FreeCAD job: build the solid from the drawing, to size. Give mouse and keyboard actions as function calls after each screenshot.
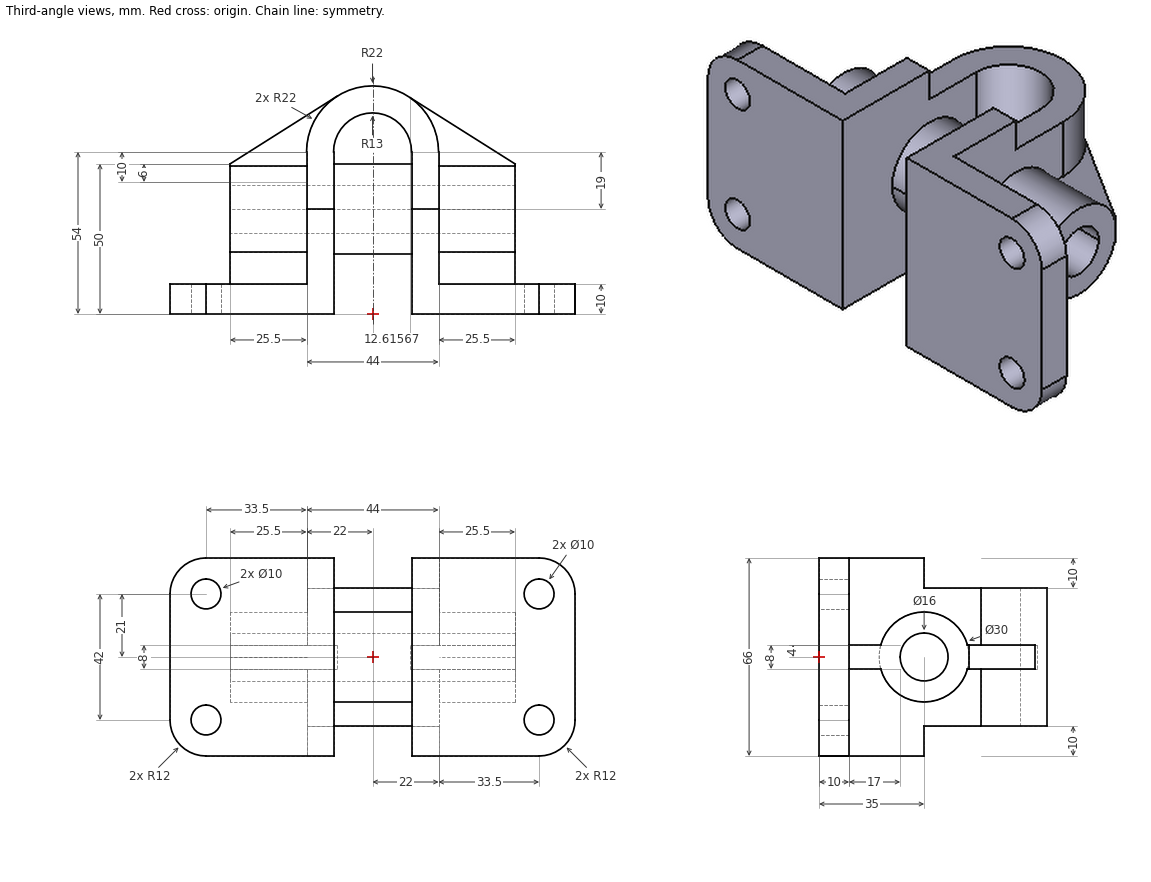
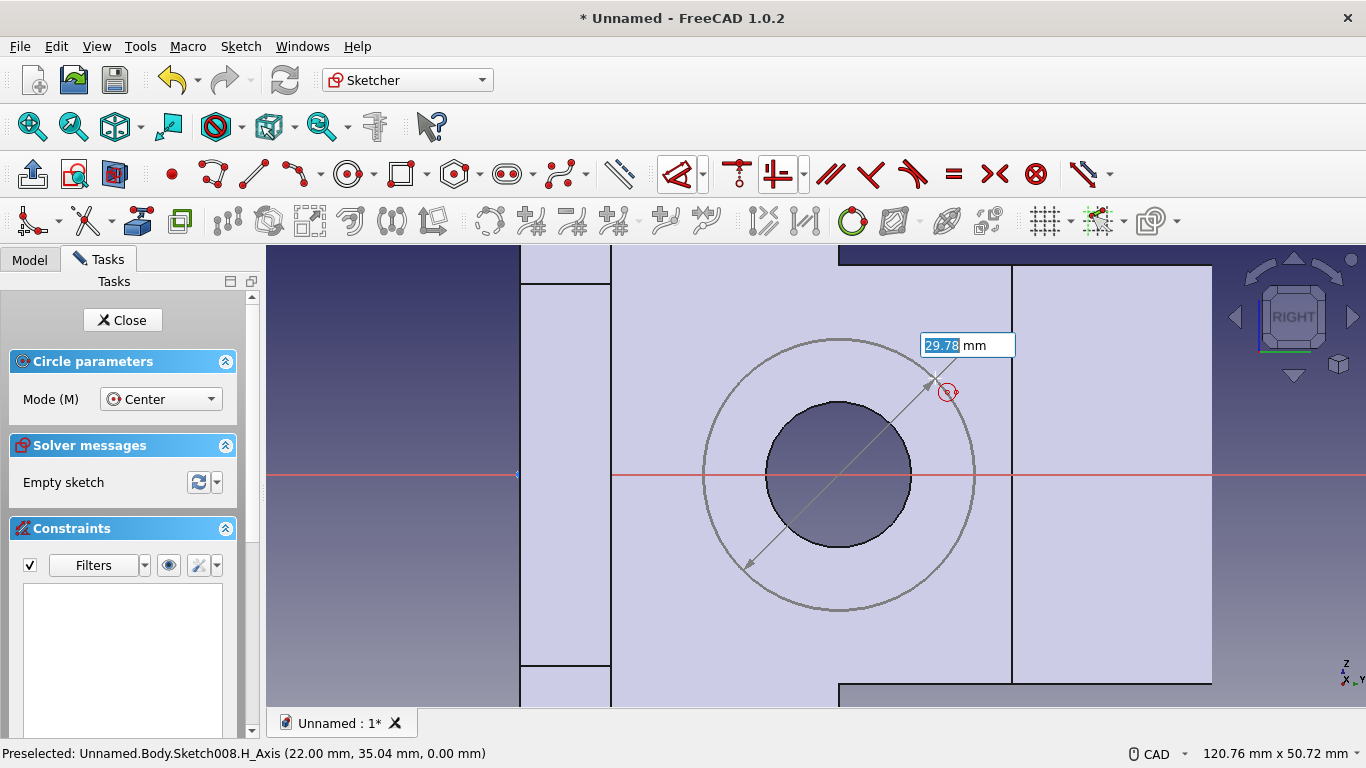
text(30)
key(Return)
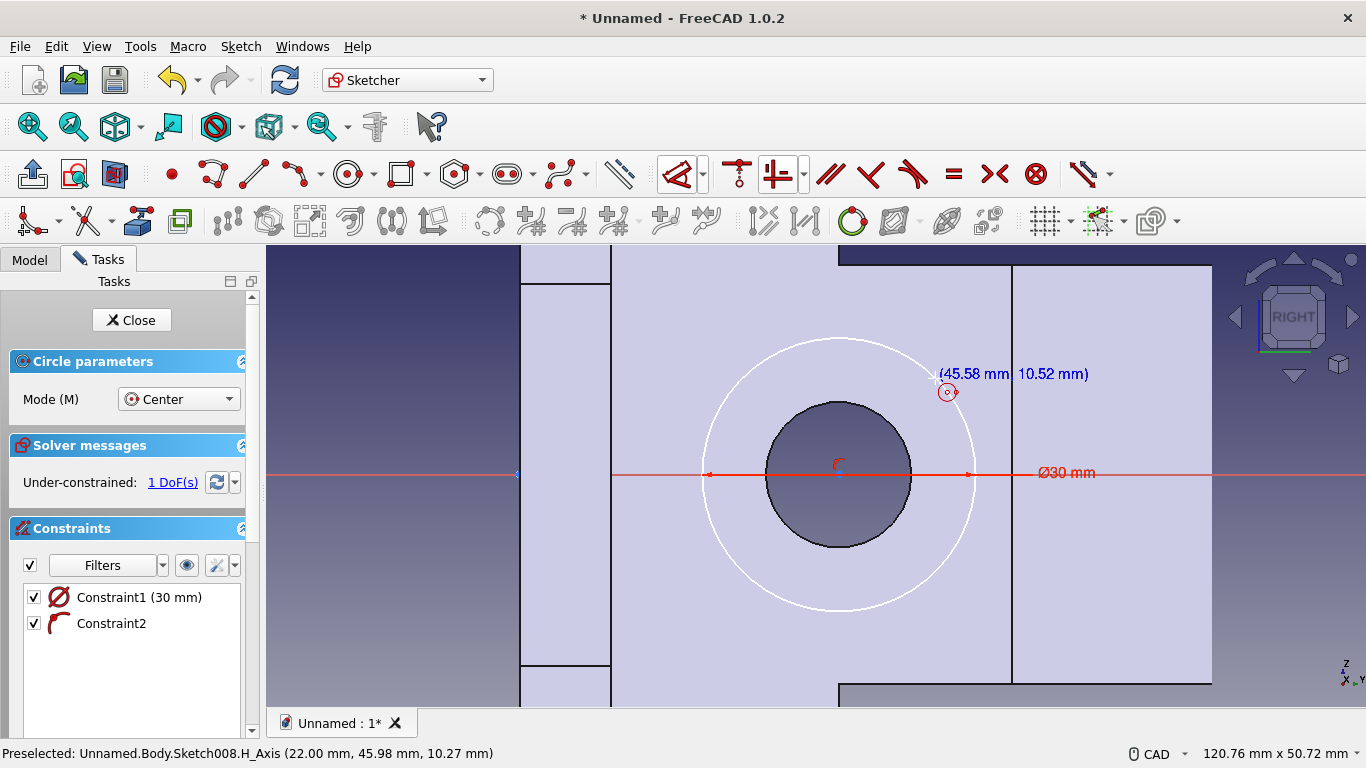
click(839, 475)
move(890, 423)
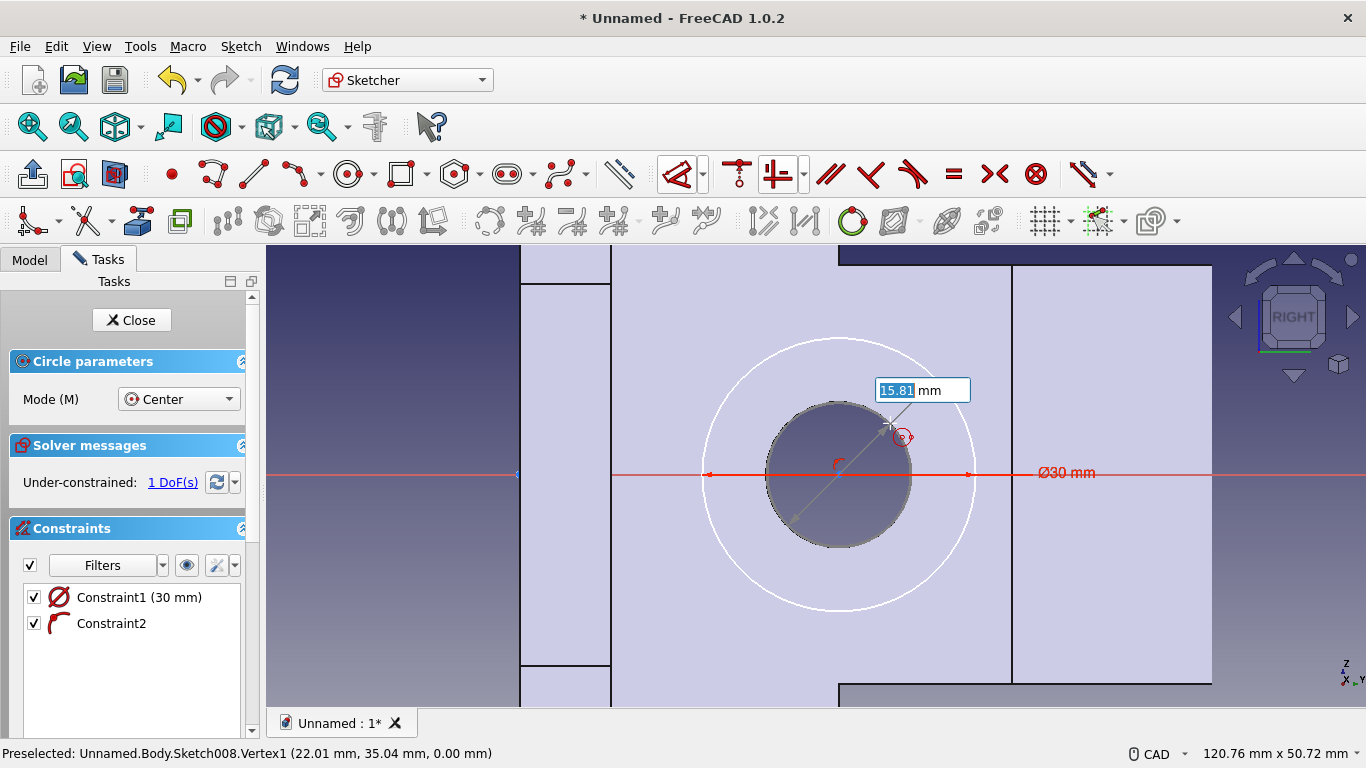
text(16)
key(Return)
key(Escape)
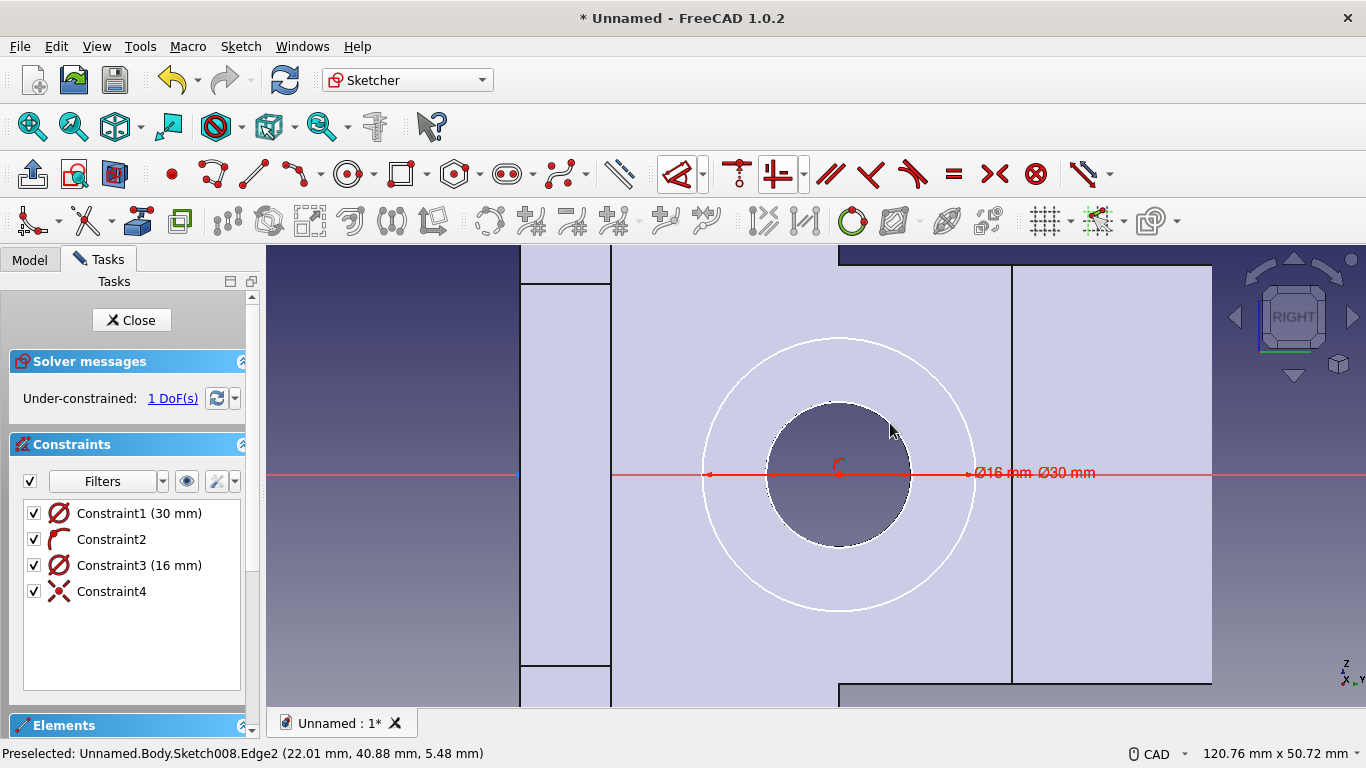
click(839, 475)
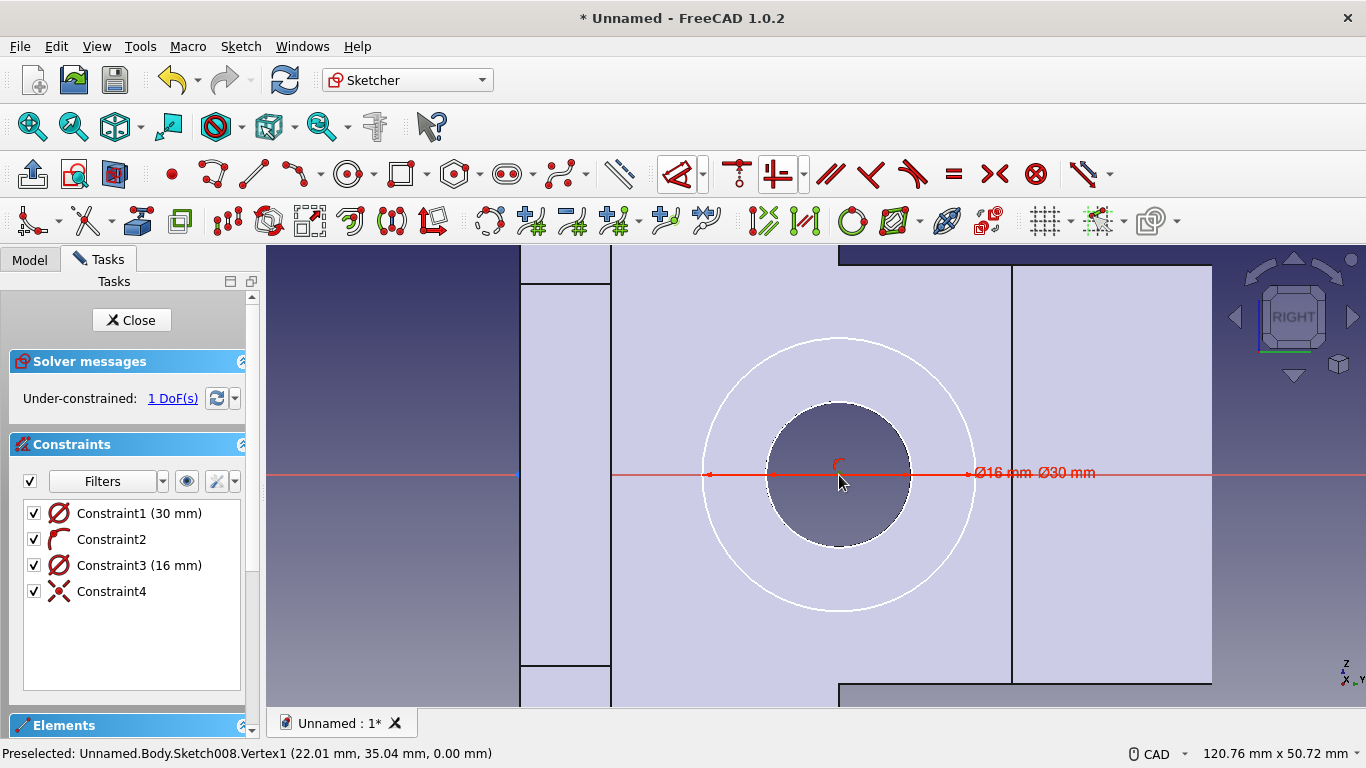
key(l)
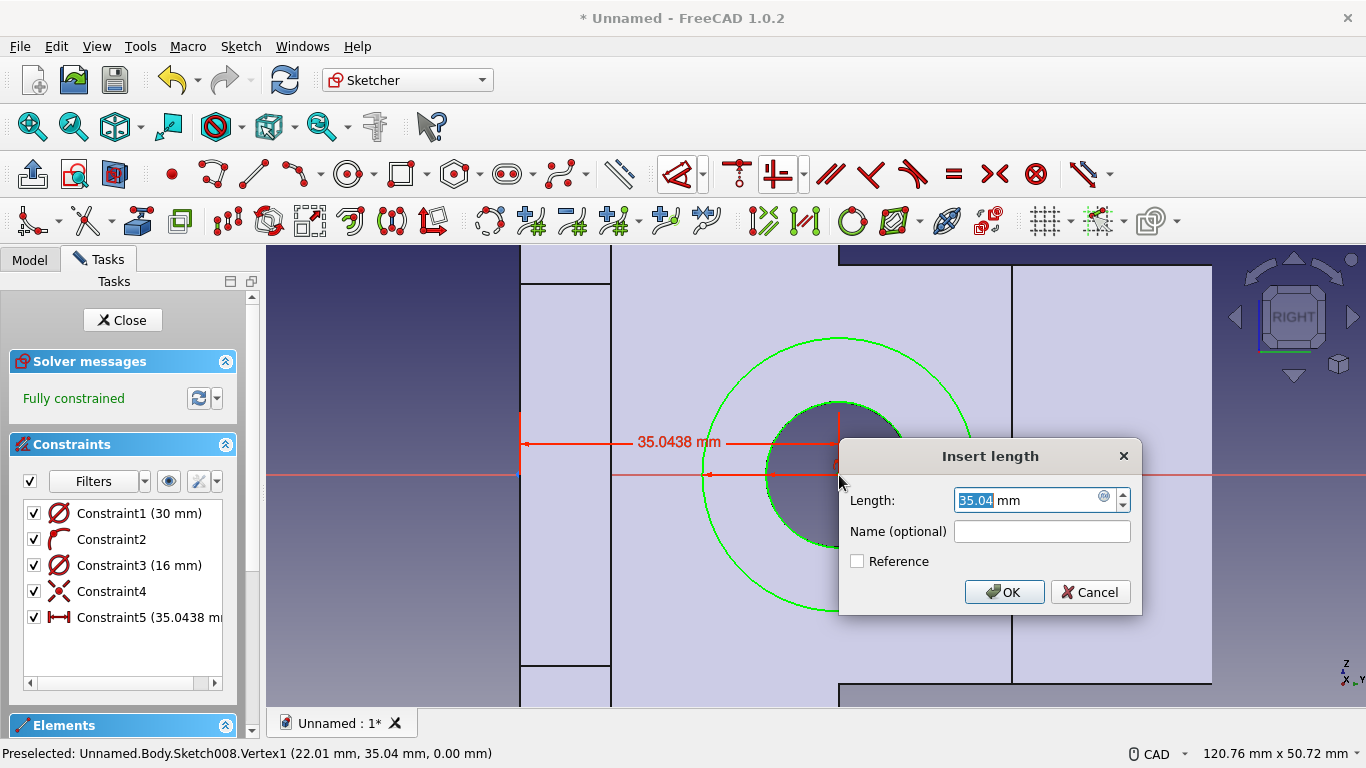
text(35)
key(Return)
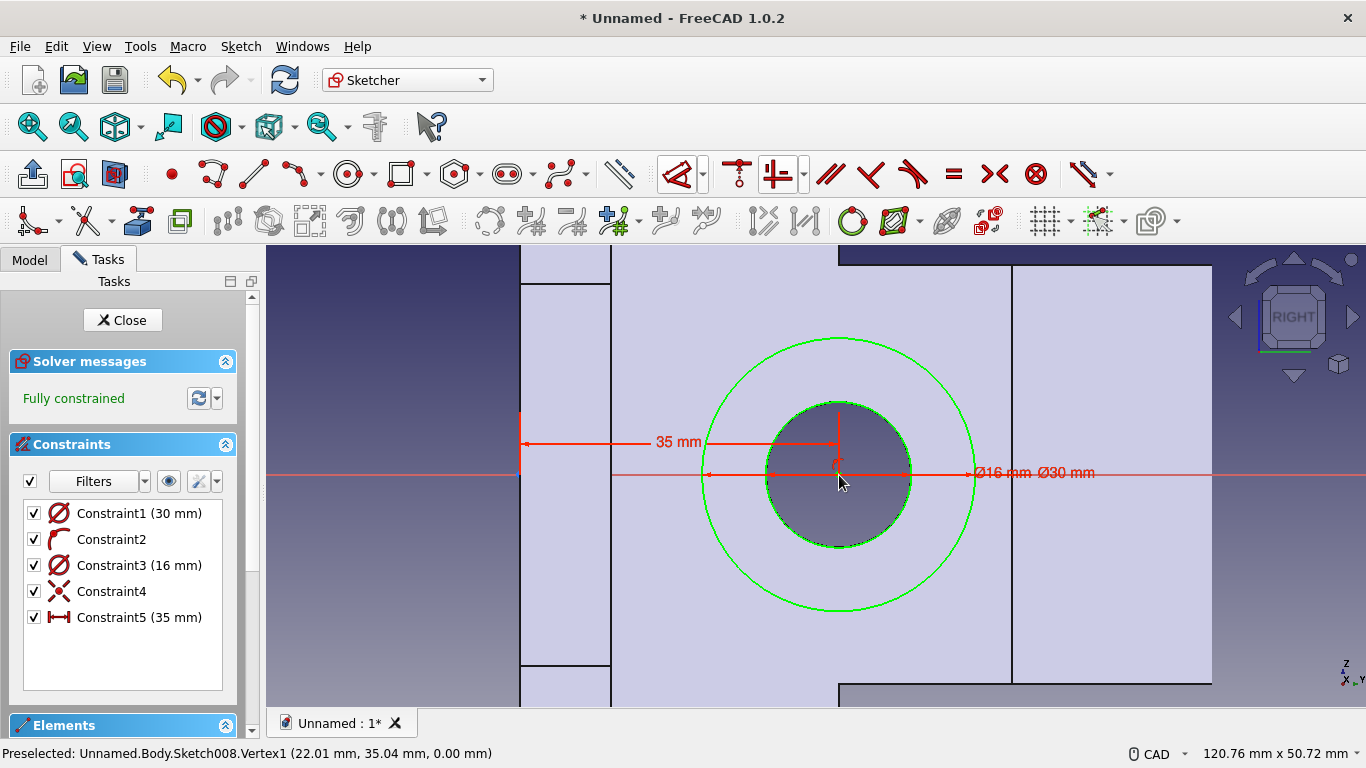
click(123, 320)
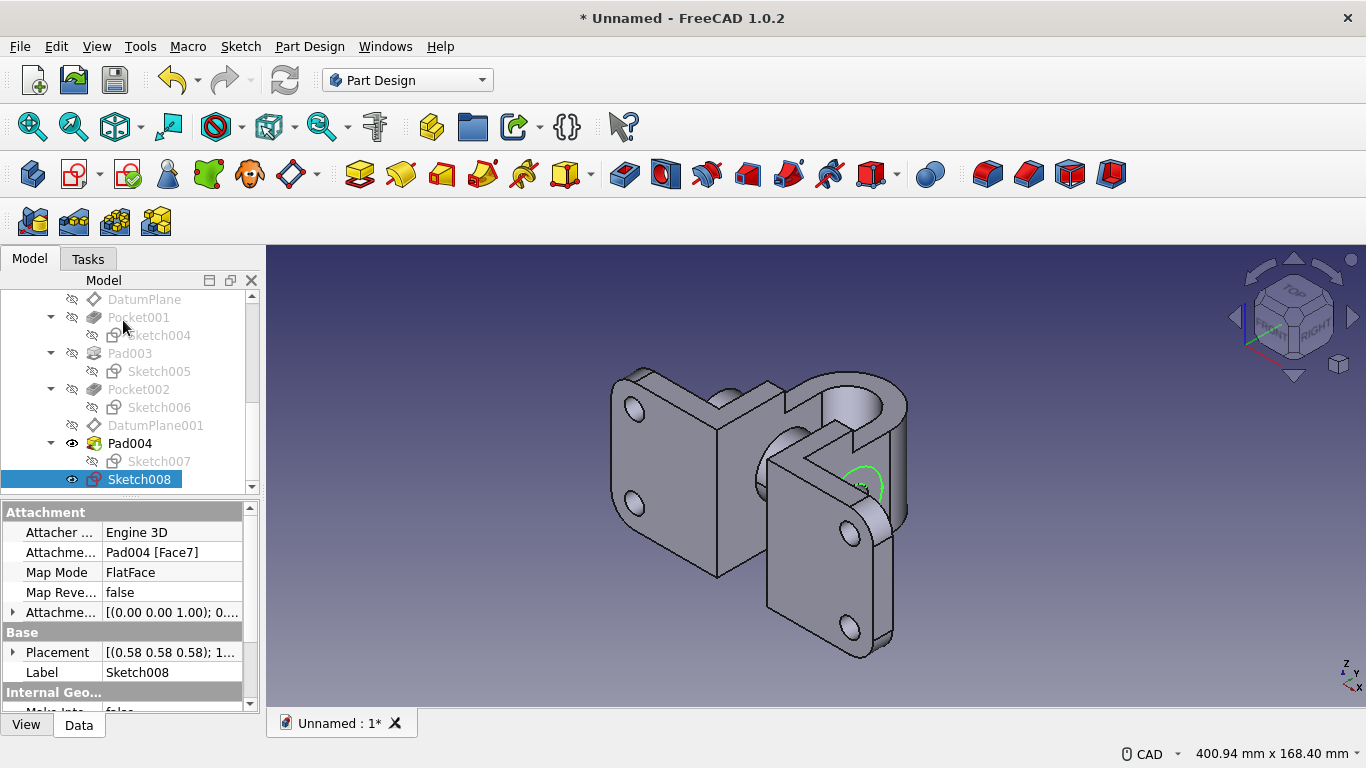
click(360, 174)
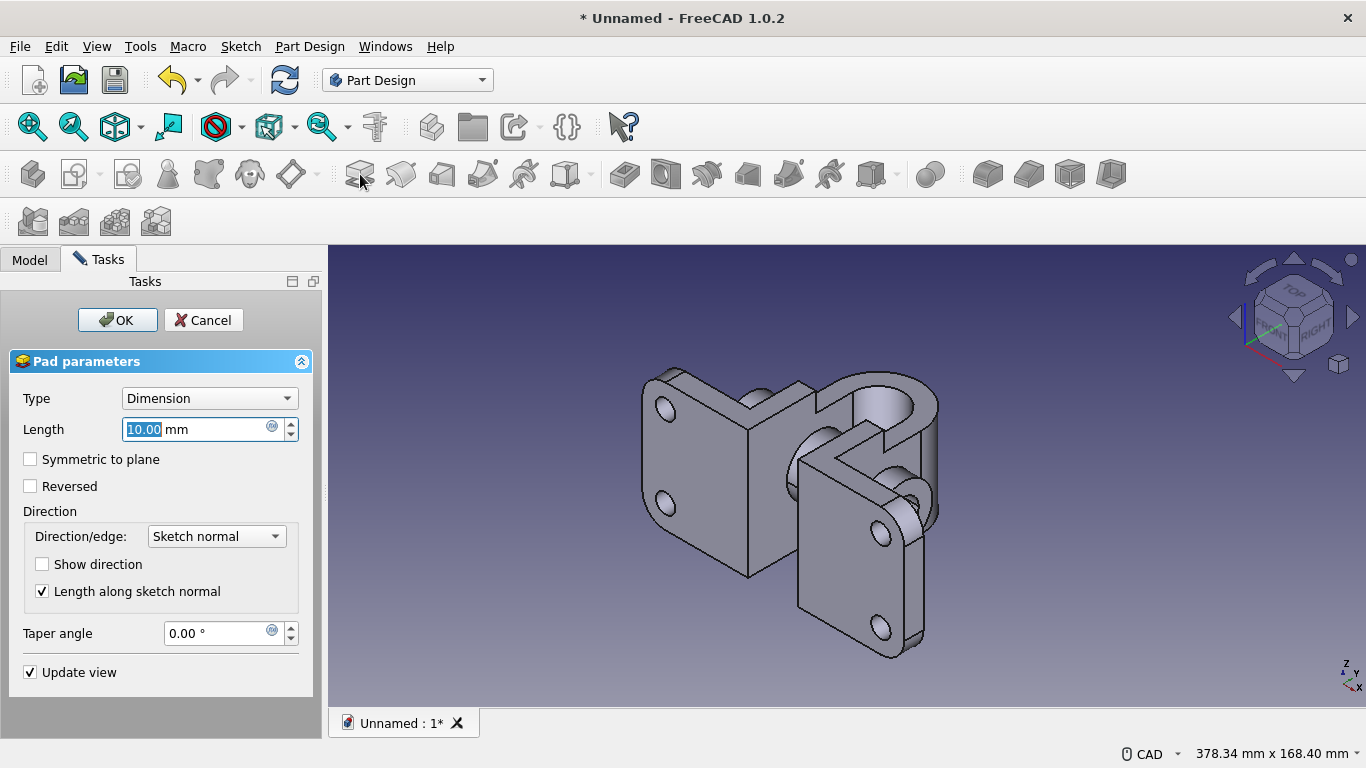
text(25.5)
key(Tab)